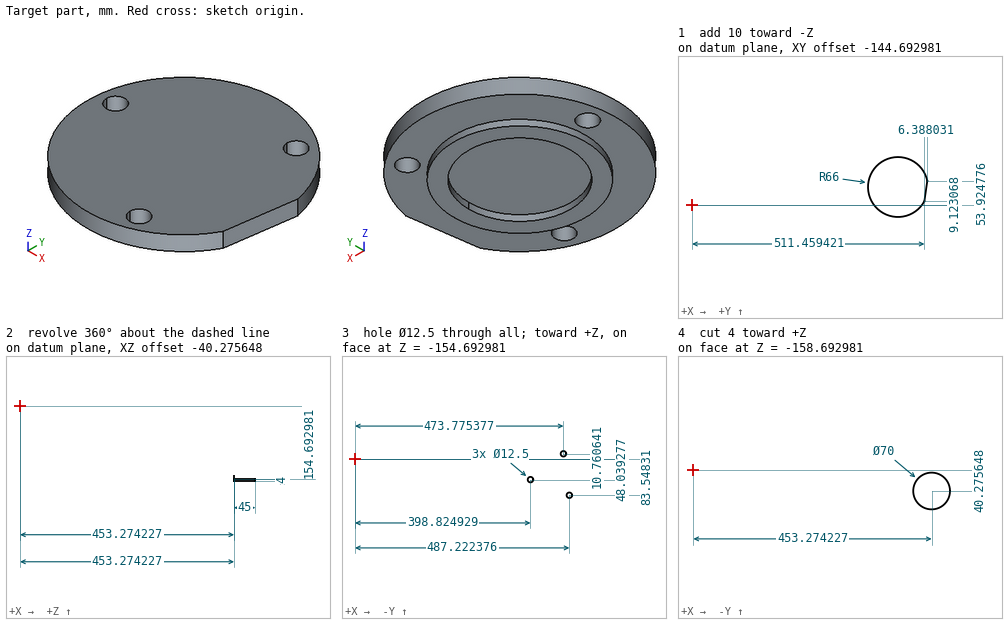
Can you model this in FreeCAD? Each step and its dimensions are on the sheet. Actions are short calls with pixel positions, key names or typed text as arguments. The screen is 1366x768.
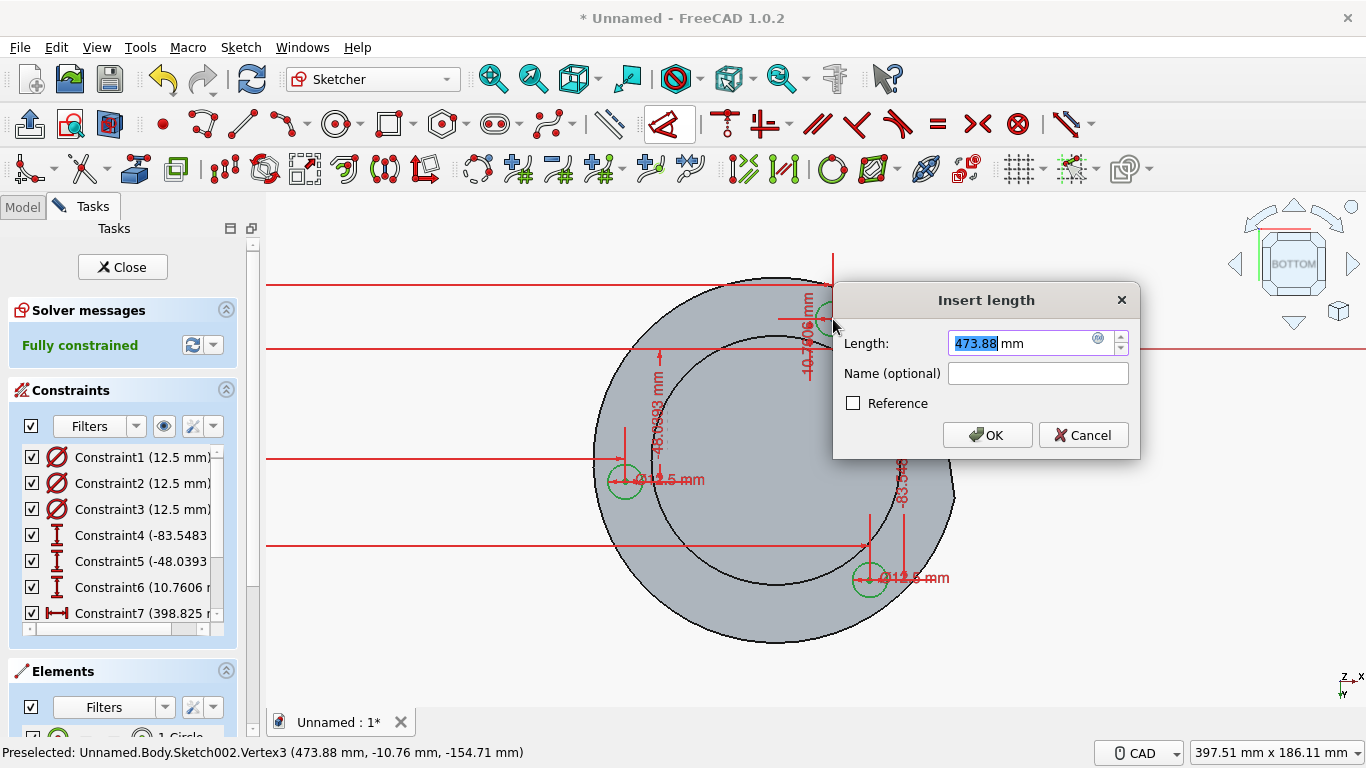
text(473.775377)
key(Return)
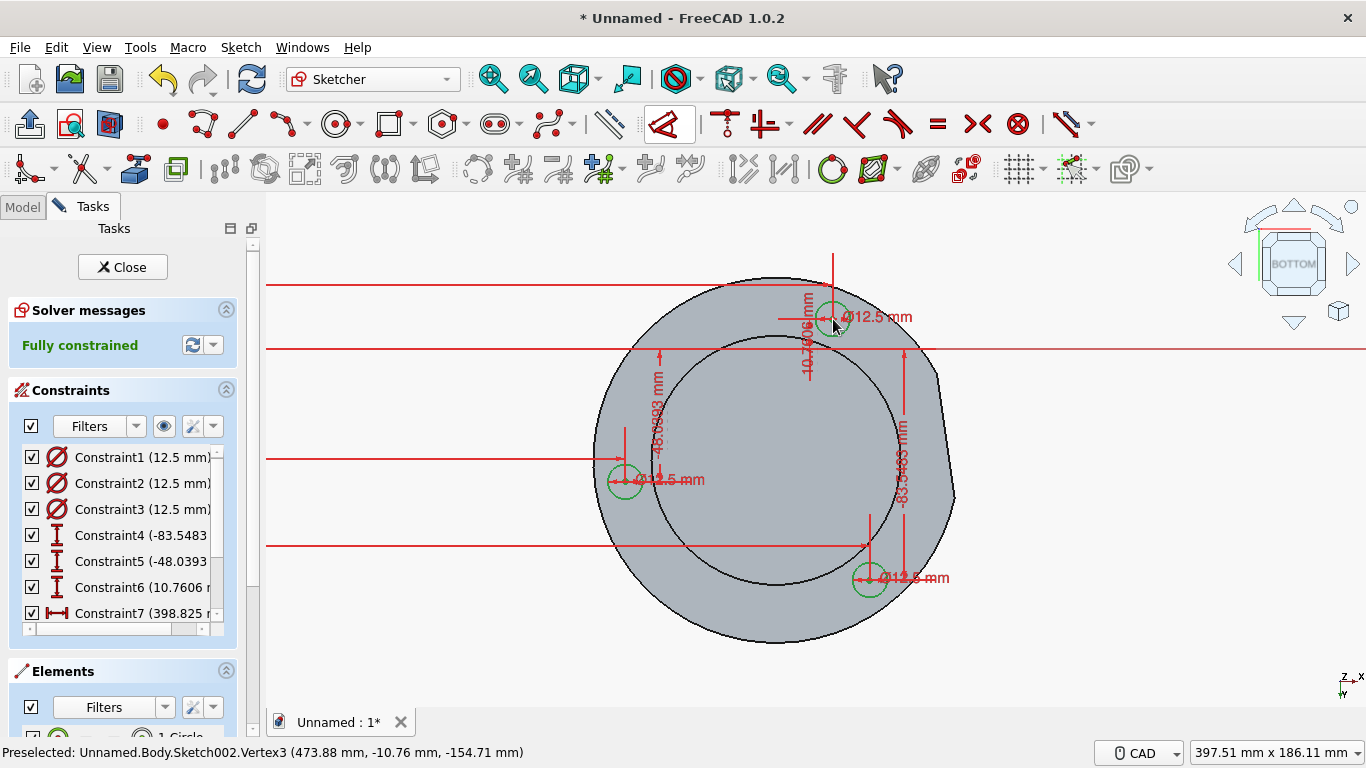
click(123, 267)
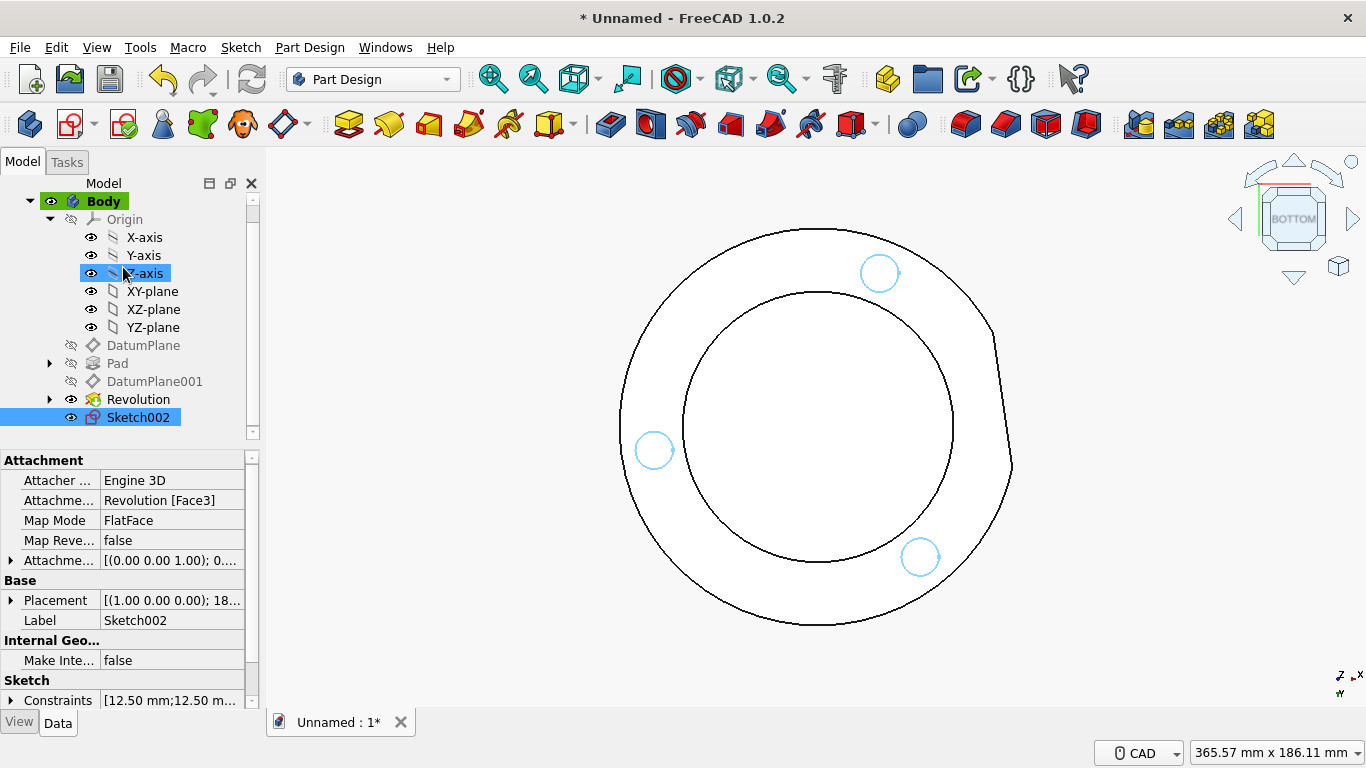
click(652, 124)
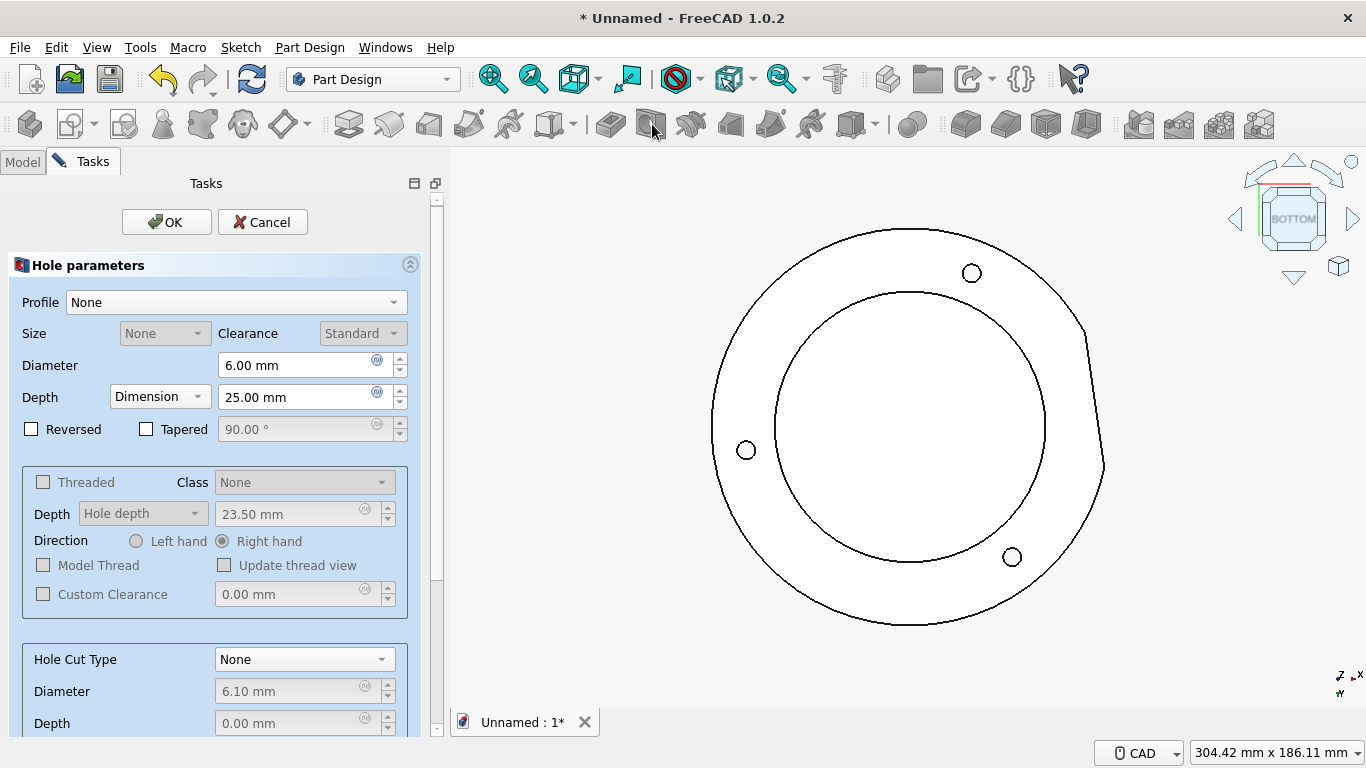
triple_click(305, 365)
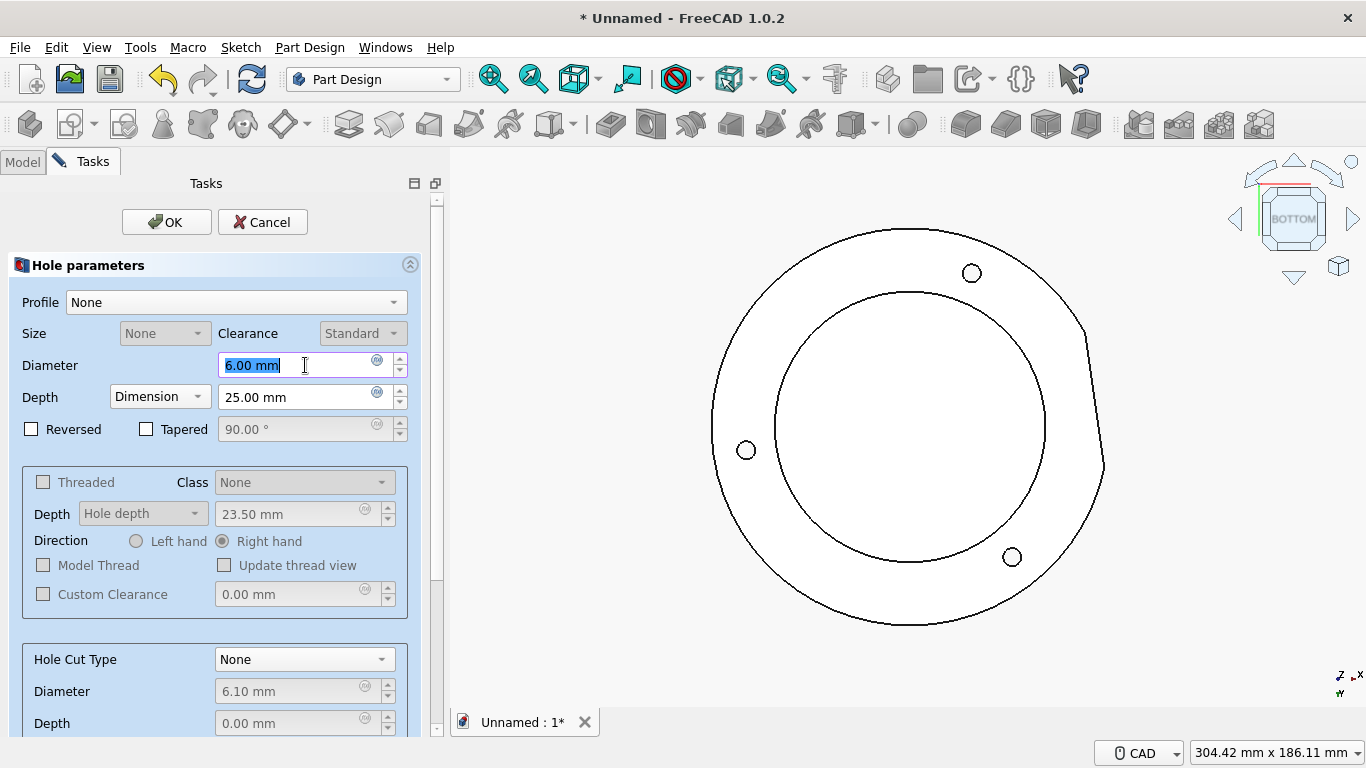
text(12.5)
key(Tab)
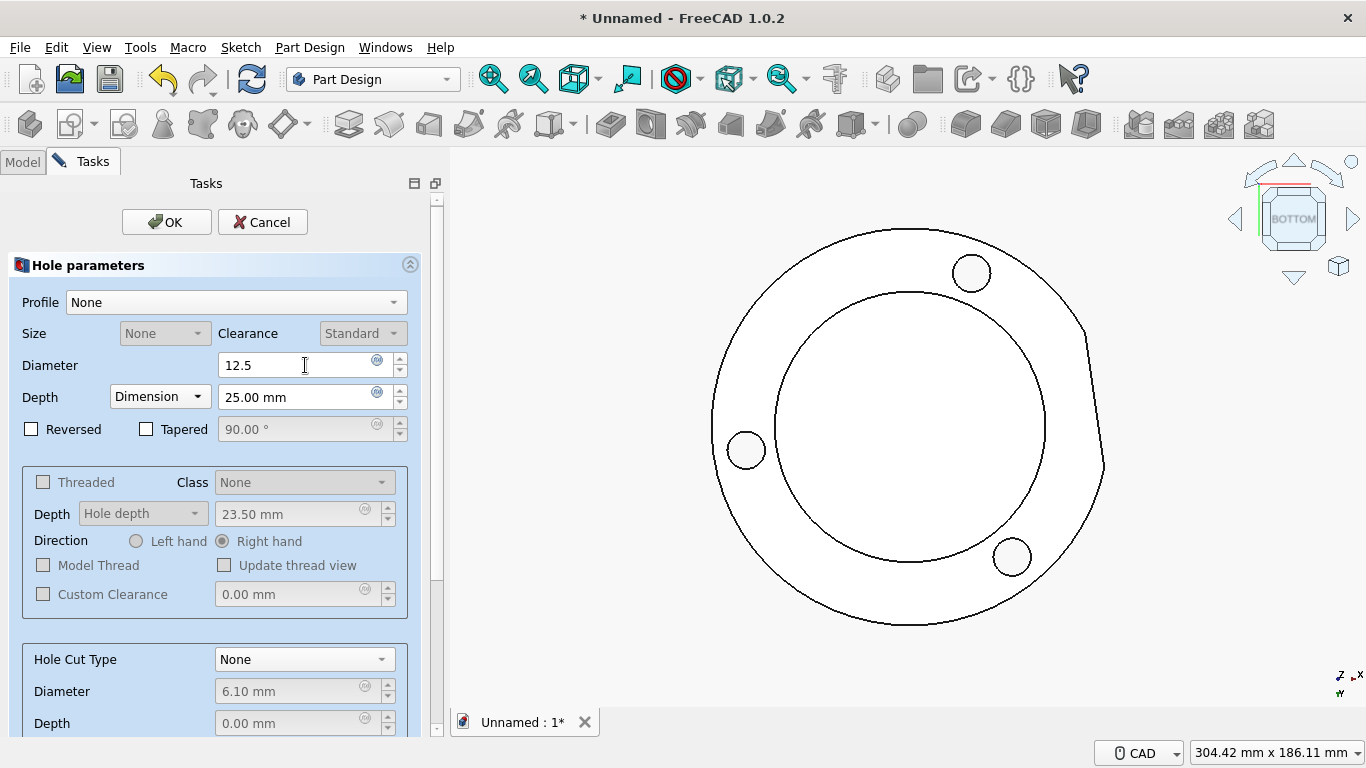
click(161, 396)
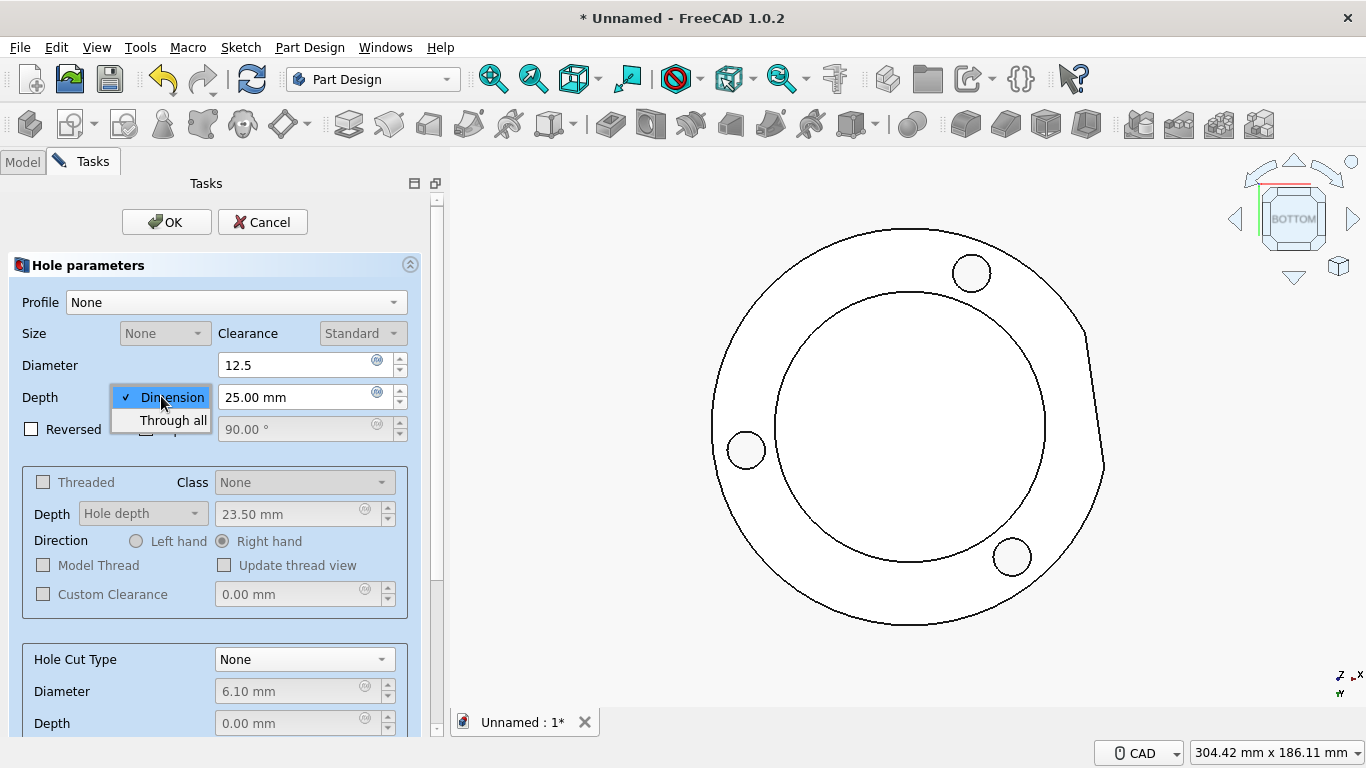
click(160, 420)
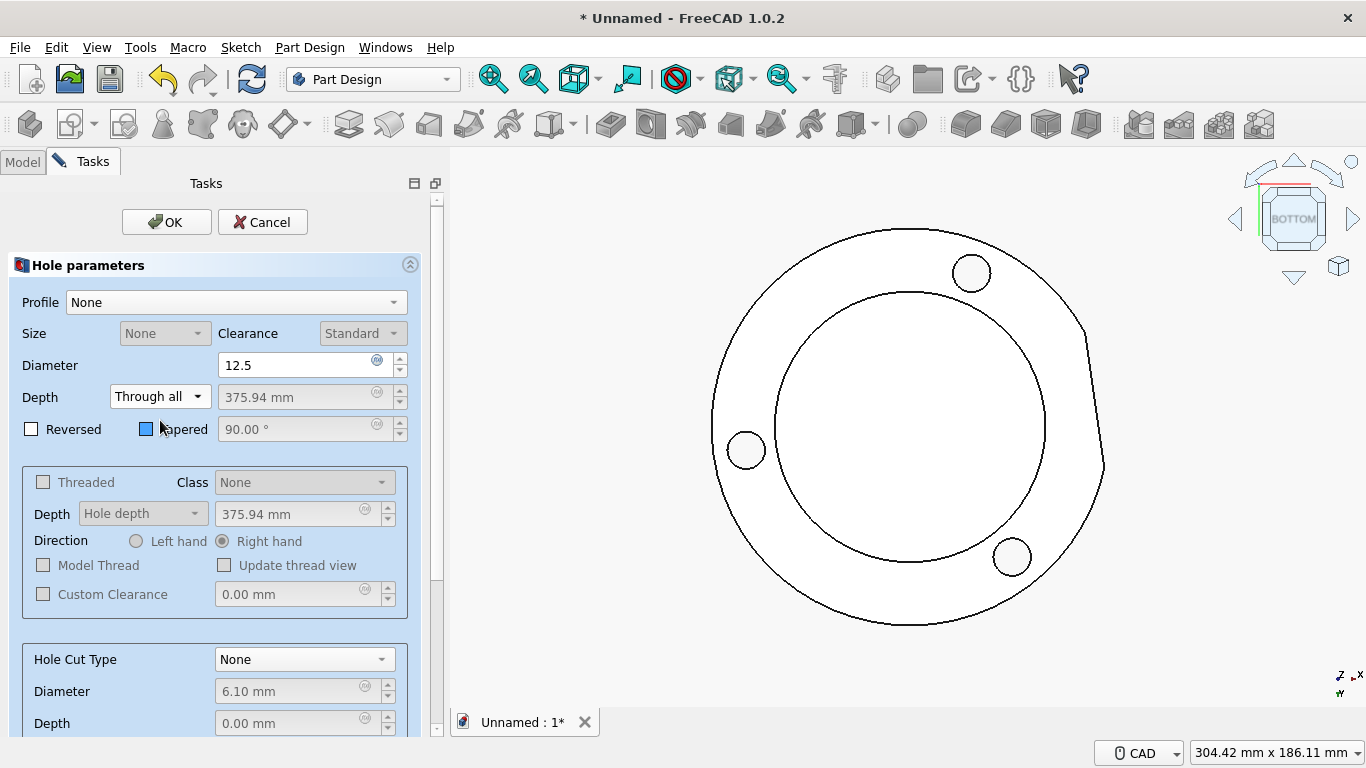
click(167, 222)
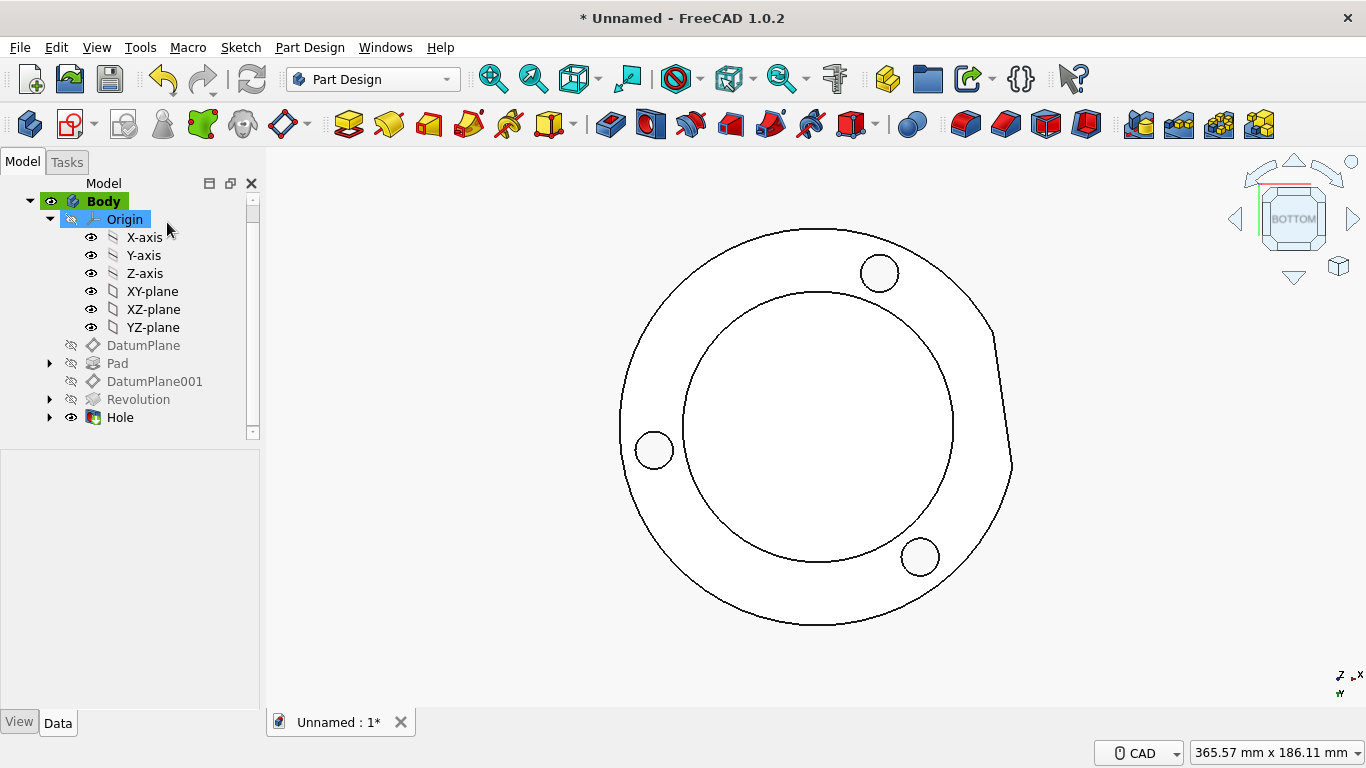
click(818, 426)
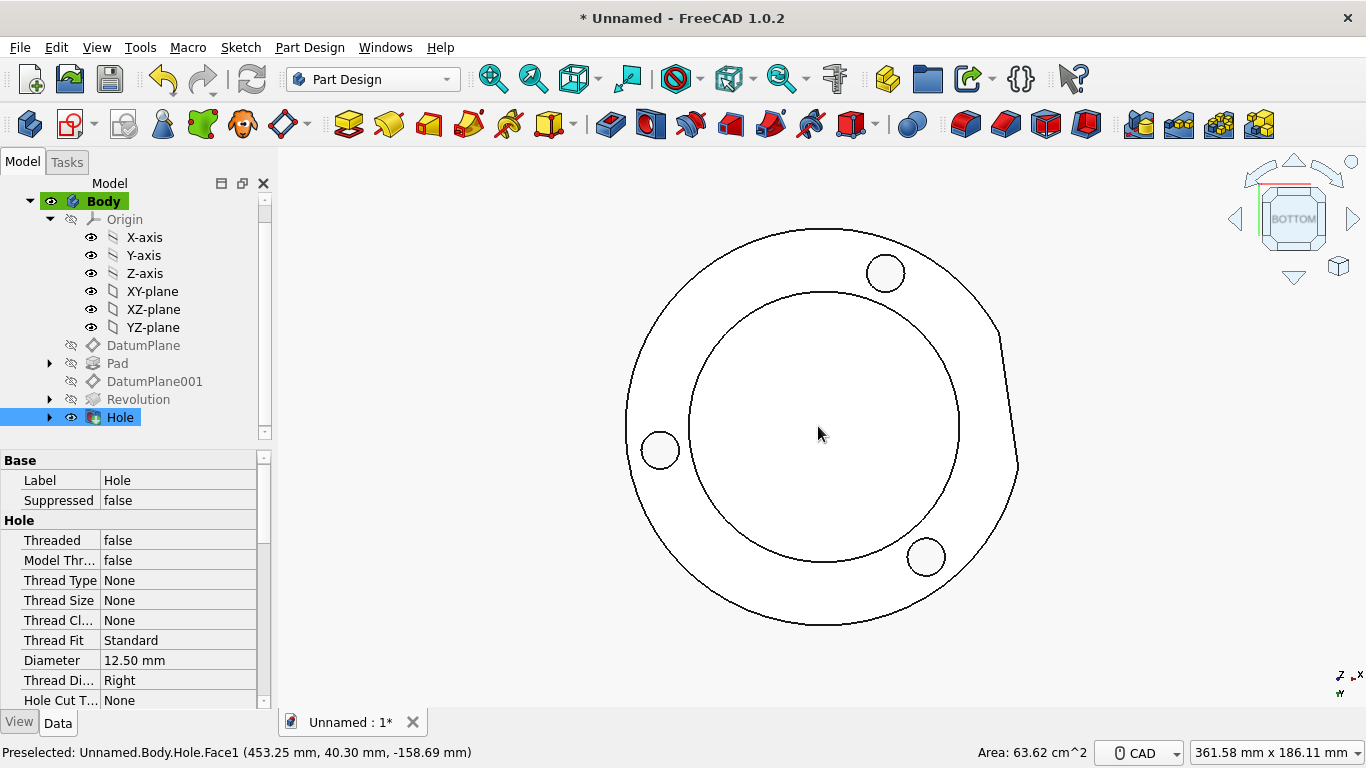
click(70, 124)